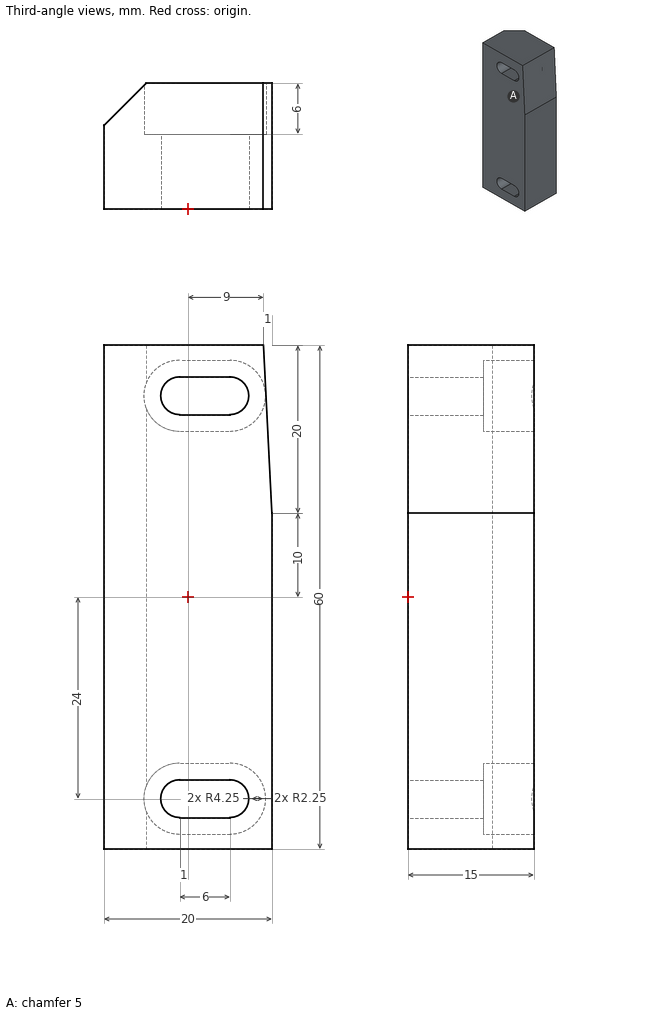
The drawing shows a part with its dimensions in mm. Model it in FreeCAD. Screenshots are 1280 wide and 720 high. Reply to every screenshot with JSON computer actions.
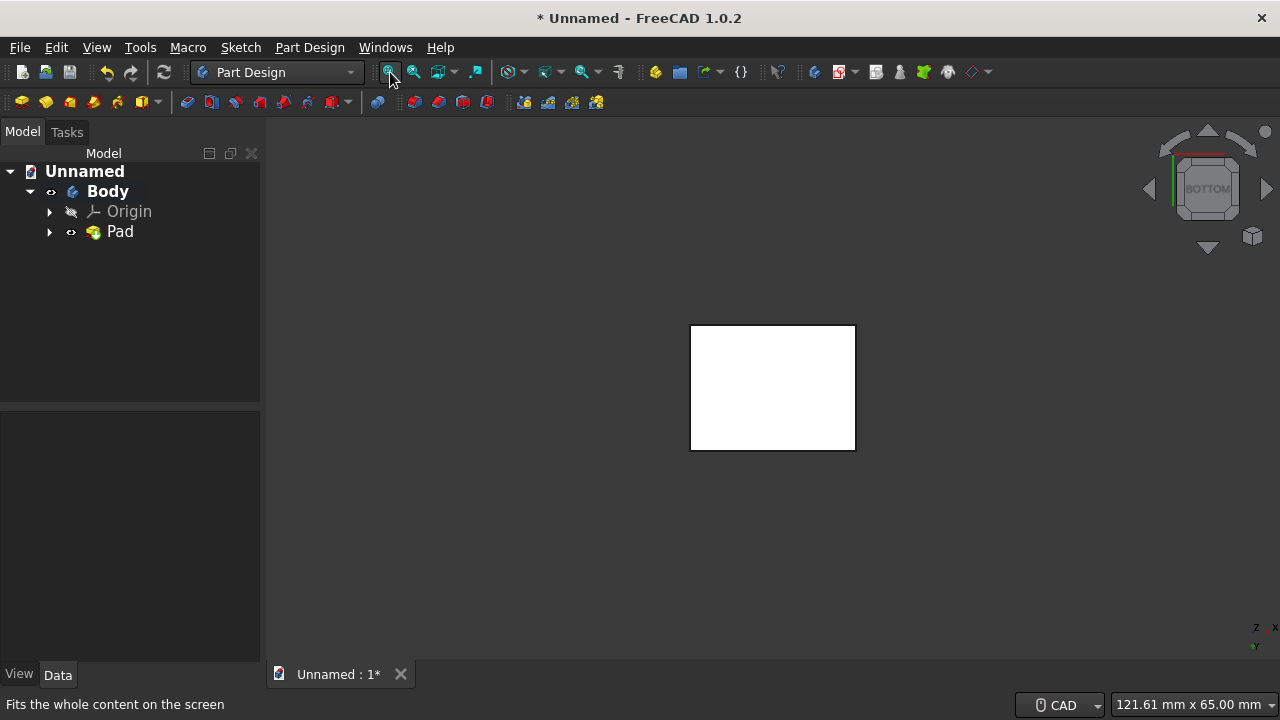
{"action": "left_click", "coordinate": [390, 72]}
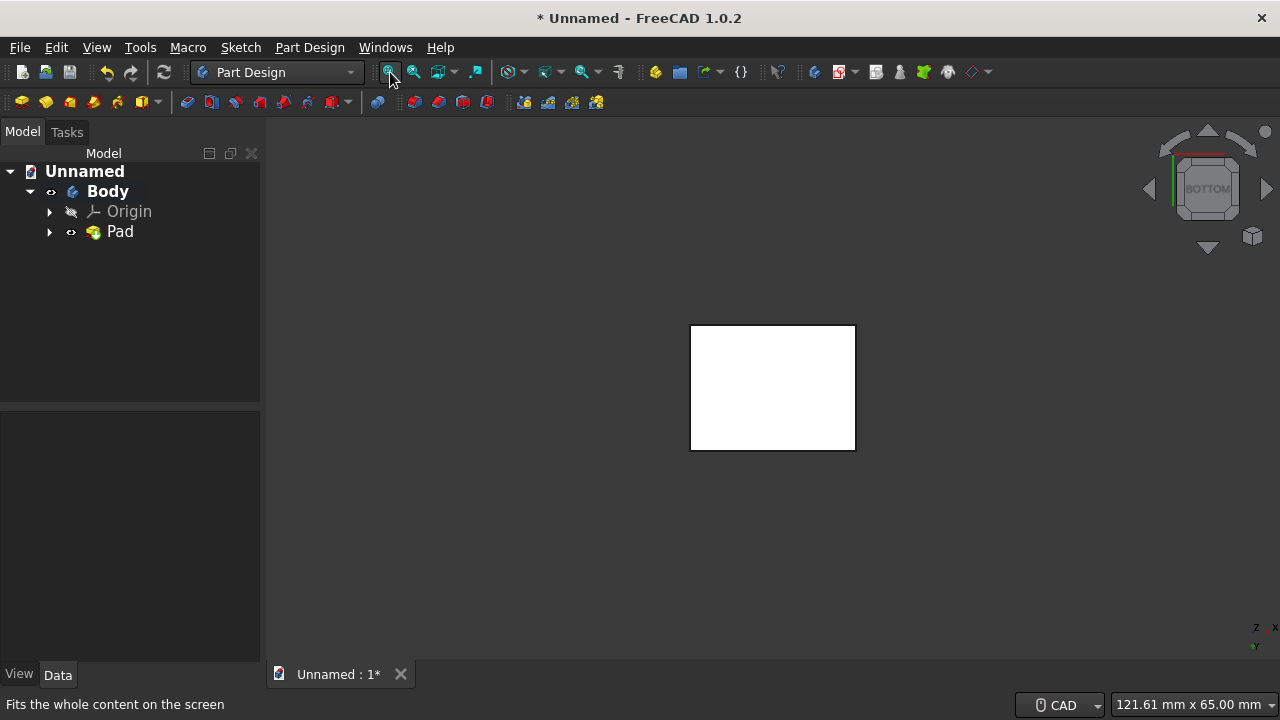
{"action": "key", "text": "4"}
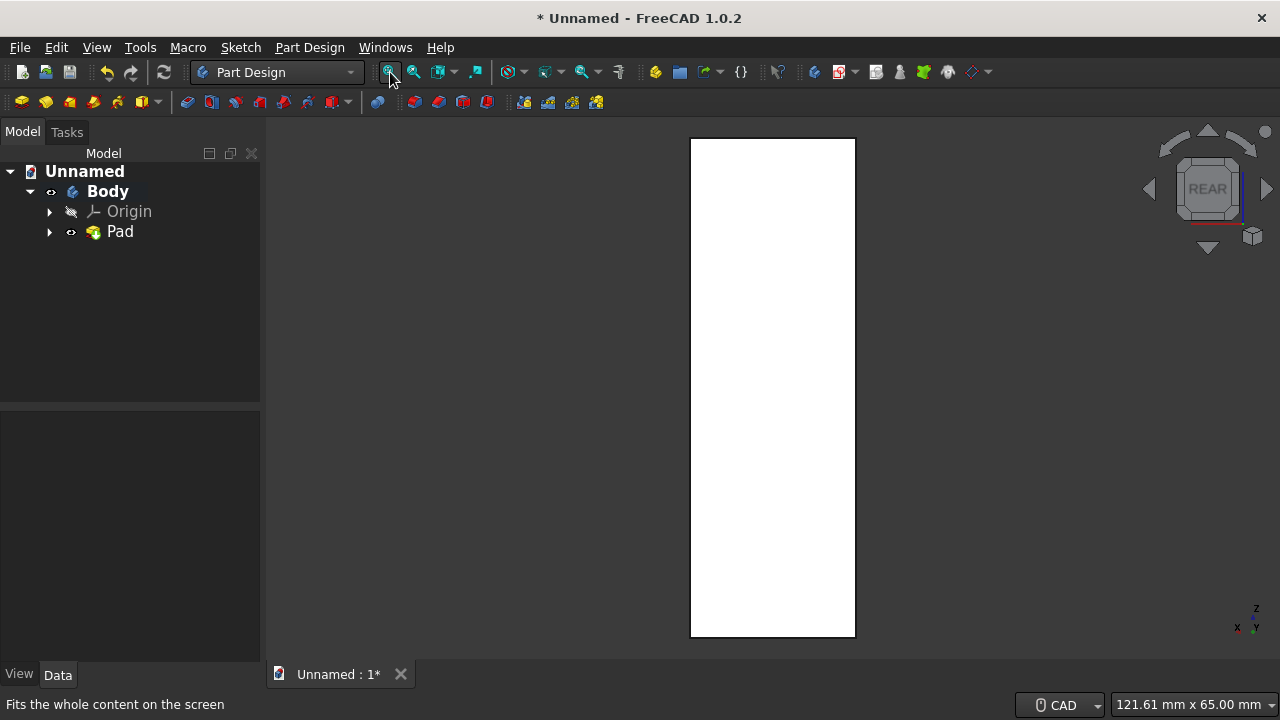
{"action": "left_click", "coordinate": [856, 387]}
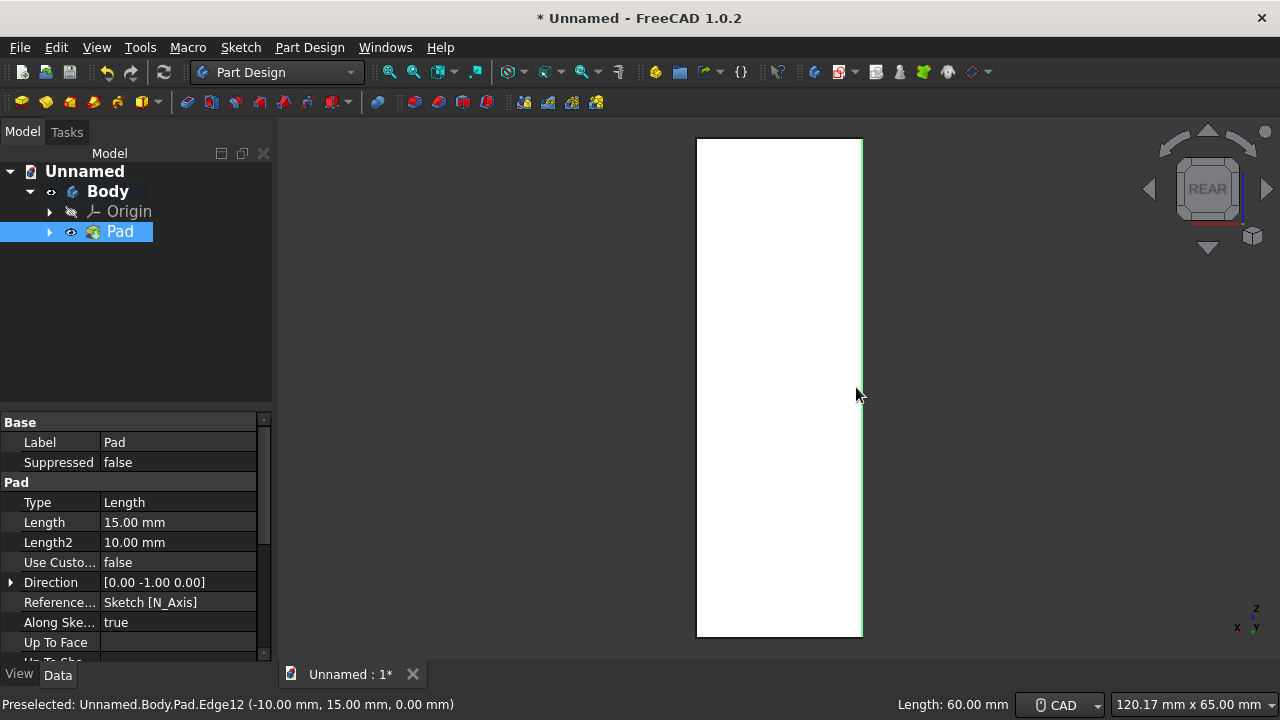
{"action": "left_click", "coordinate": [440, 102]}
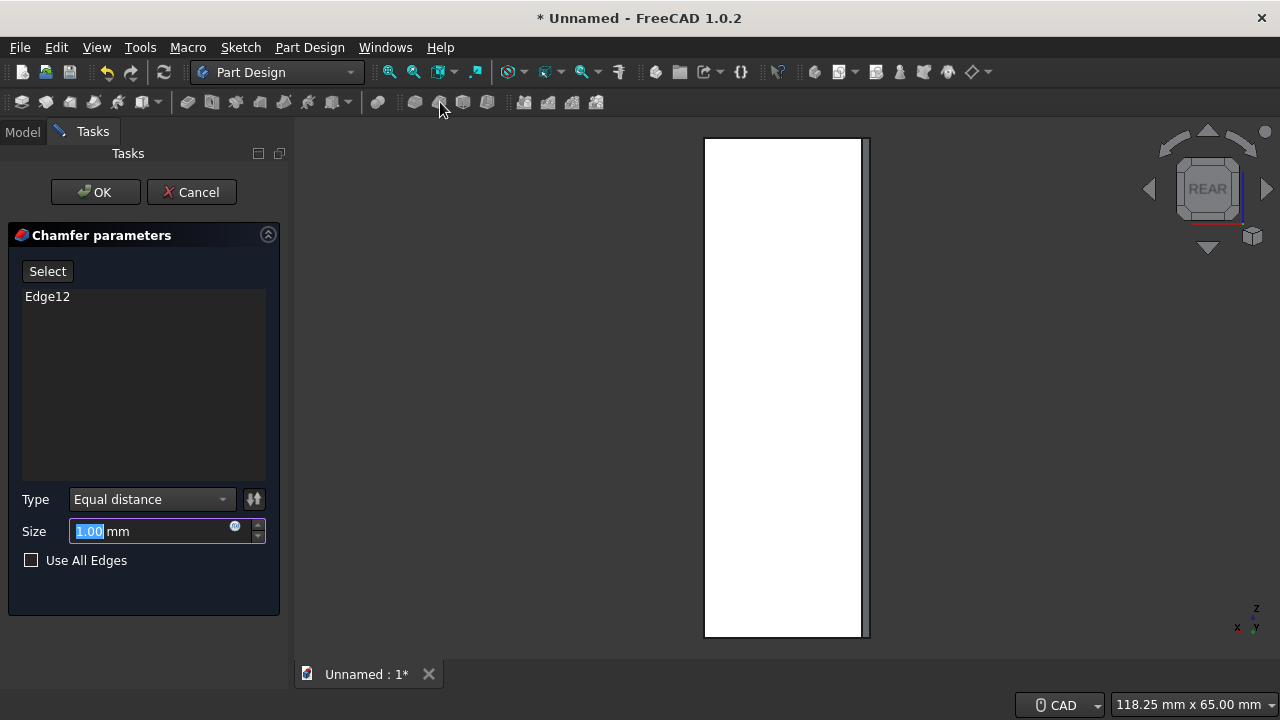
{"action": "type", "text": "5"}
{"action": "key", "text": "Tab"}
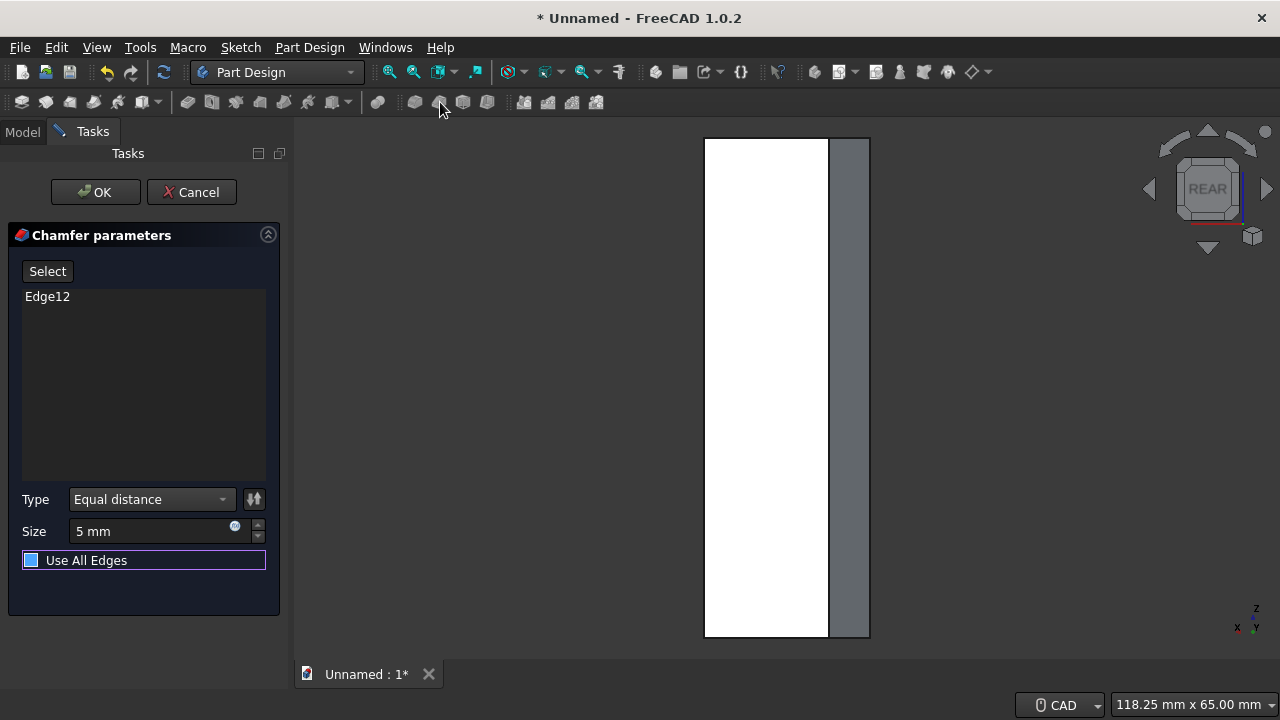
{"action": "left_click", "coordinate": [96, 192]}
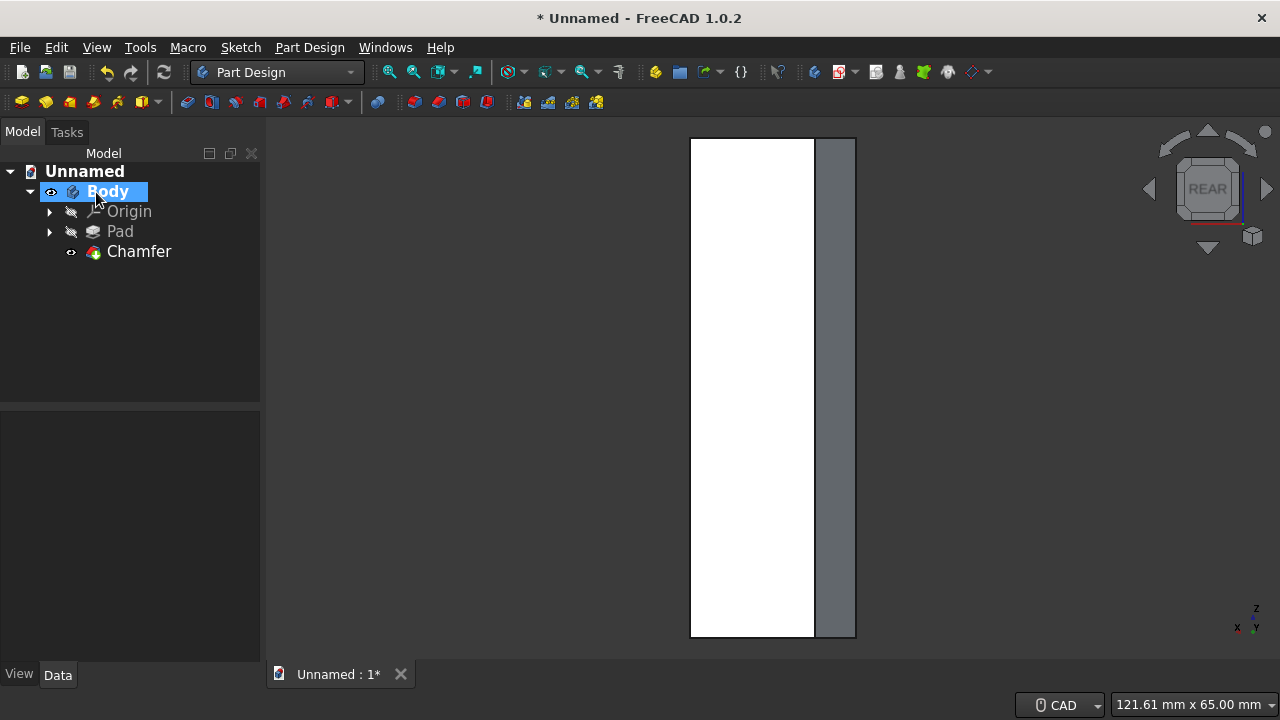
{"action": "left_click", "coordinate": [752, 244]}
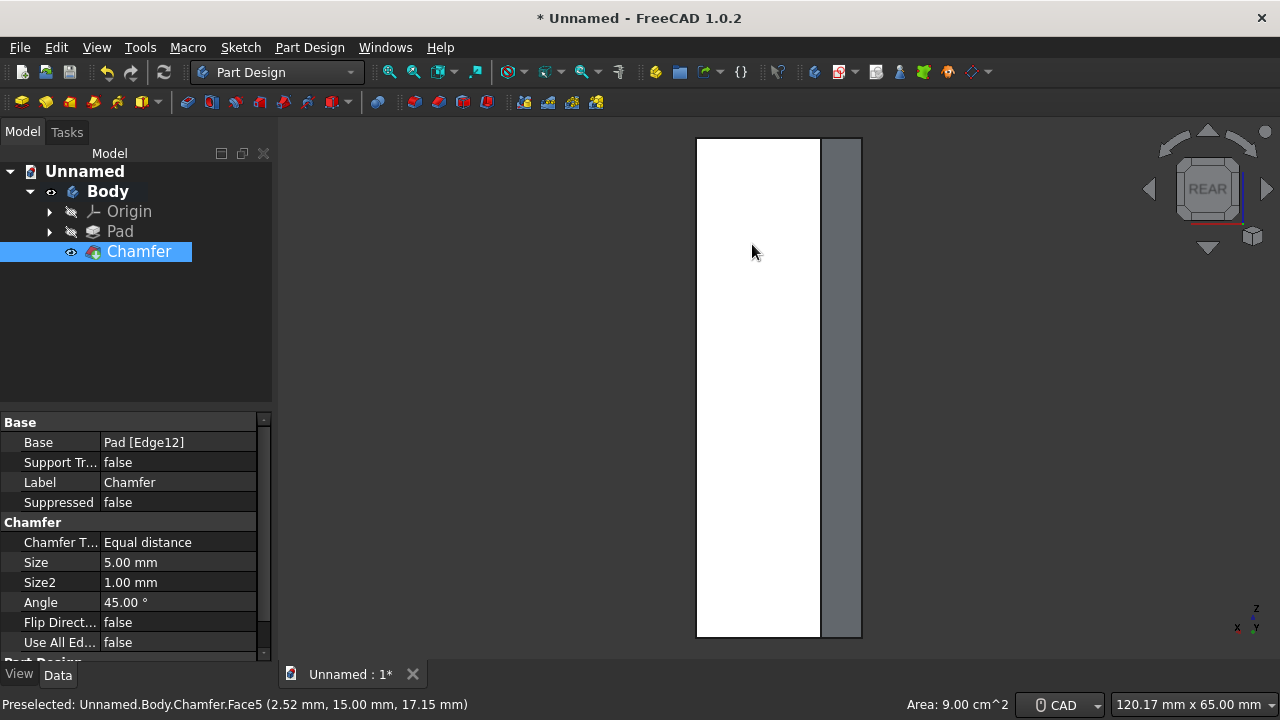
{"action": "left_click", "coordinate": [840, 72]}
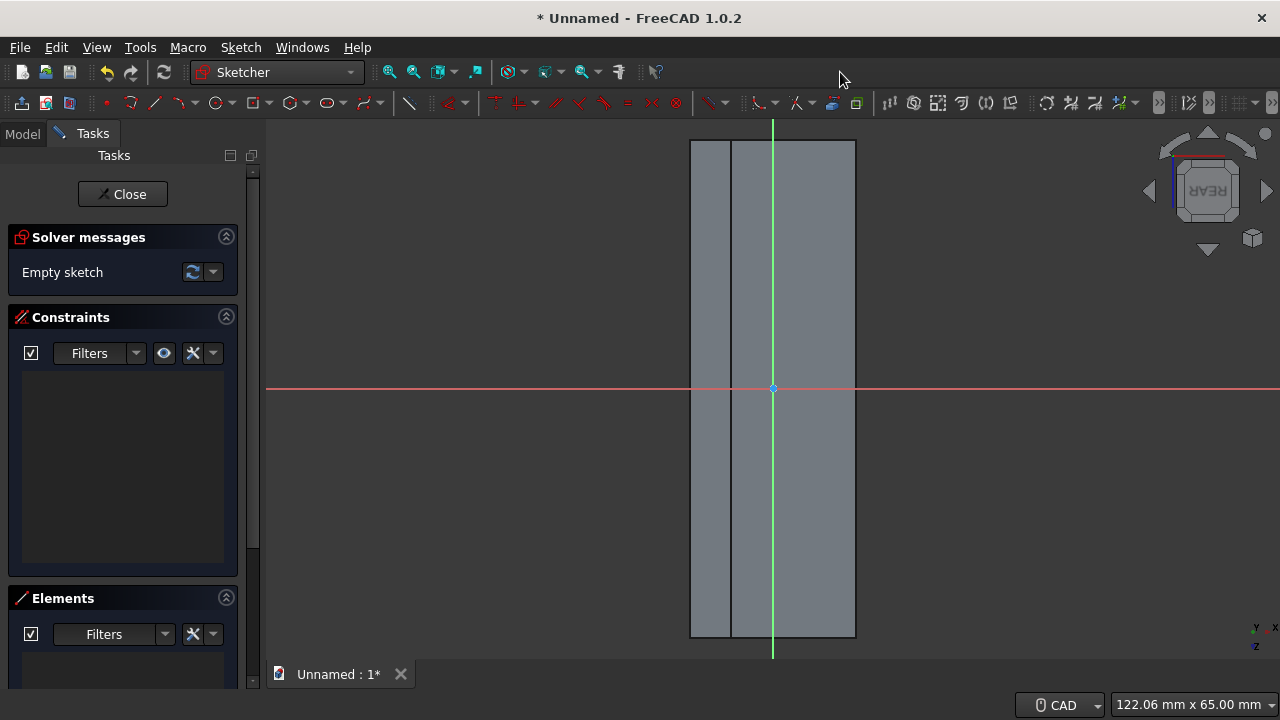
{"action": "scroll", "coordinate": [294, 147], "scroll_direction": "down", "scroll_amount": 1}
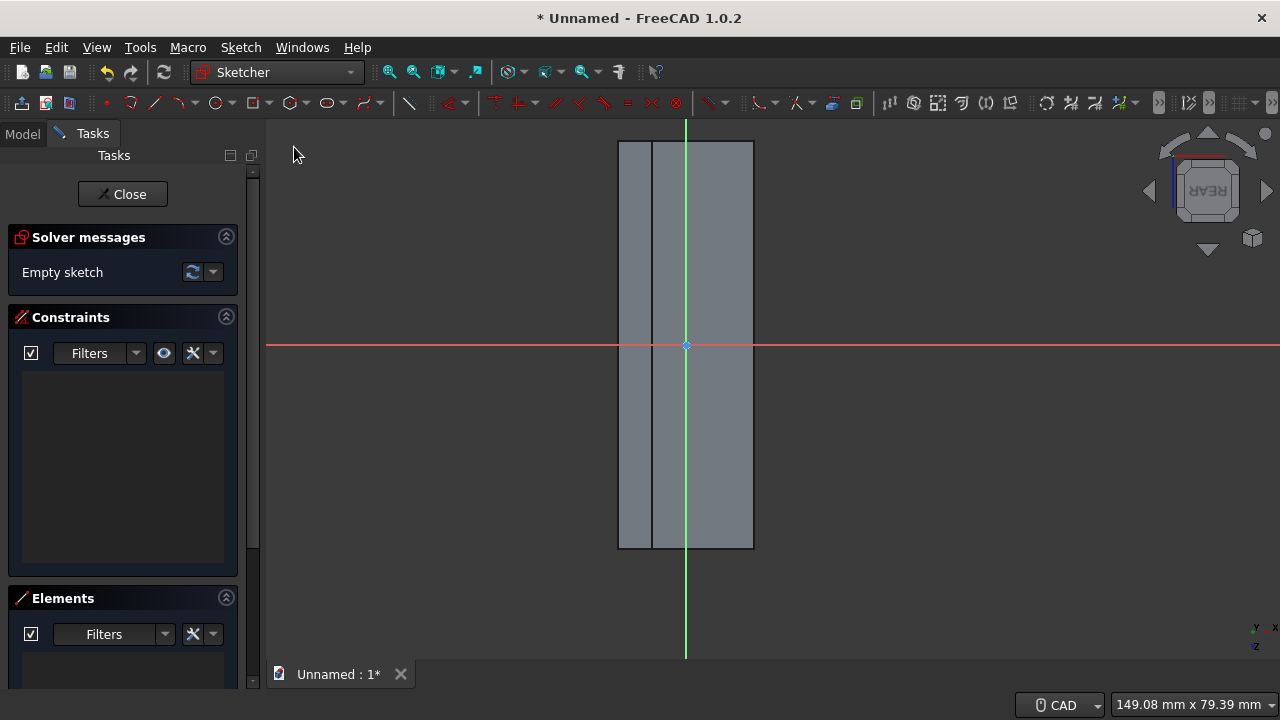
{"action": "scroll", "coordinate": [739, 518], "scroll_direction": "up", "scroll_amount": 3}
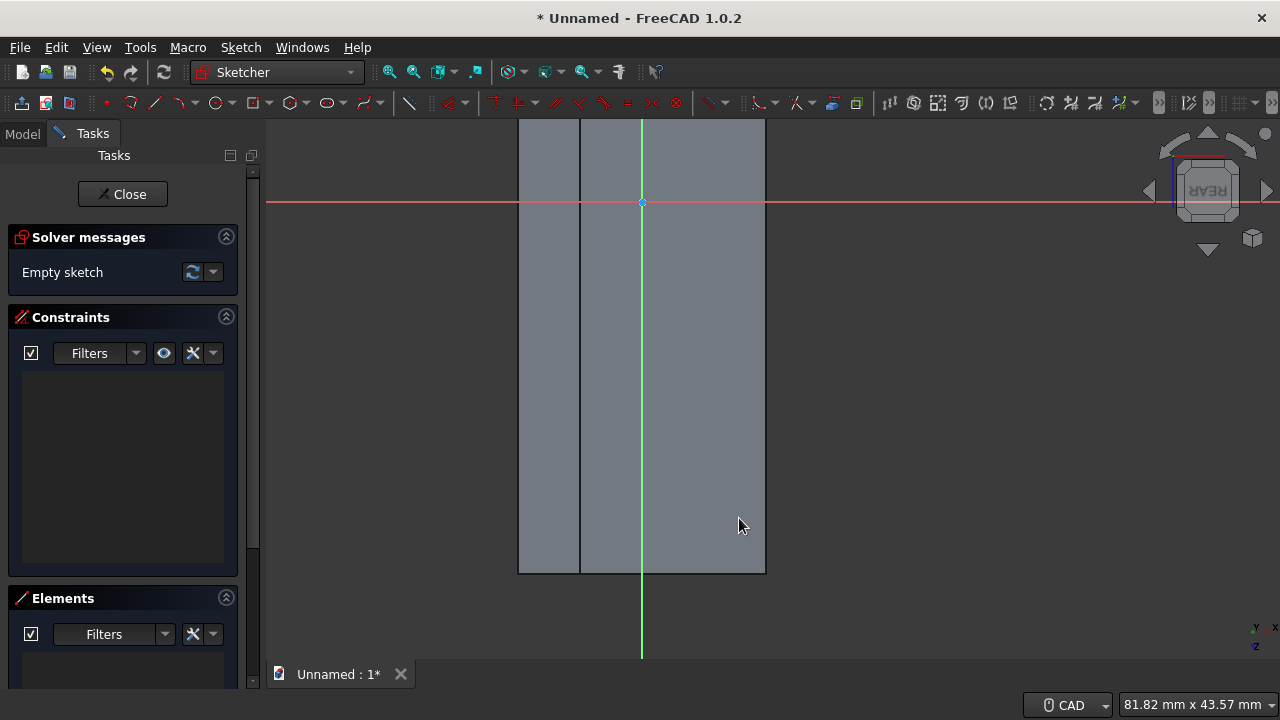
{"action": "left_click", "coordinate": [132, 104]}